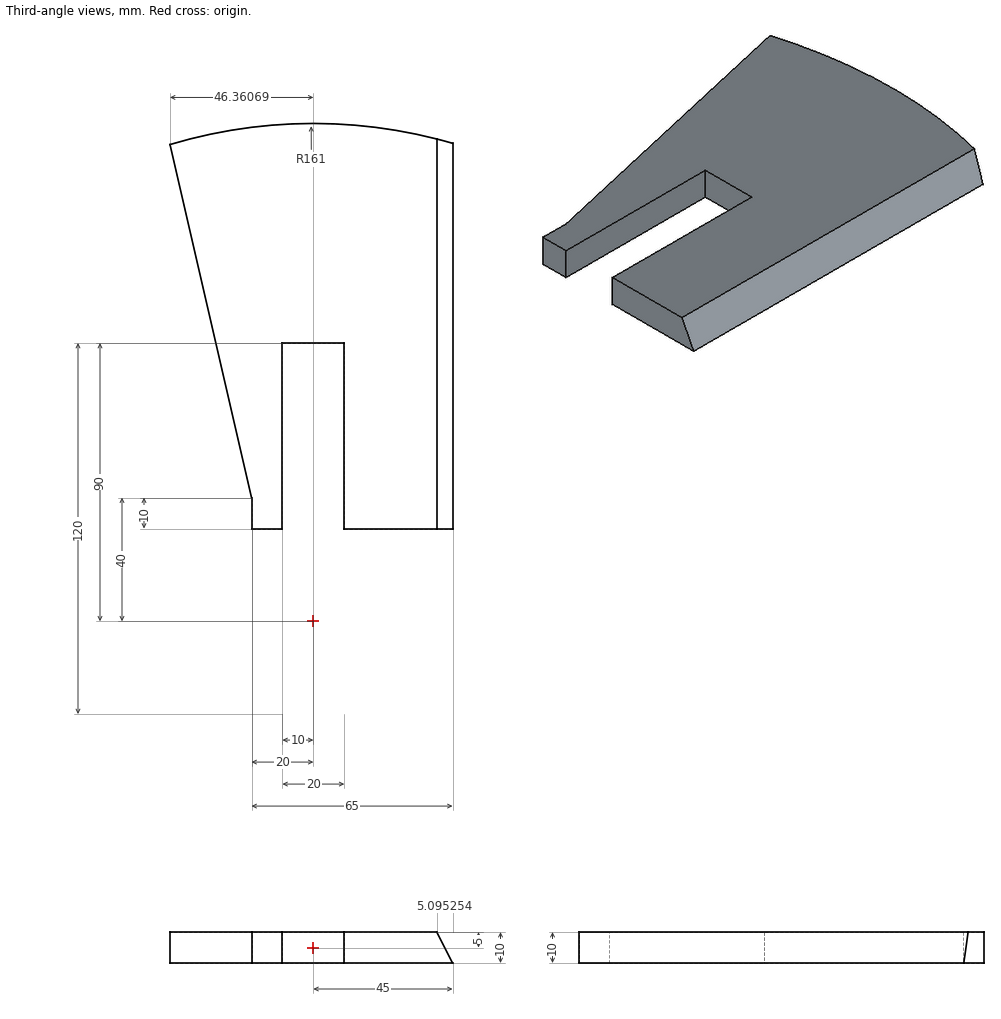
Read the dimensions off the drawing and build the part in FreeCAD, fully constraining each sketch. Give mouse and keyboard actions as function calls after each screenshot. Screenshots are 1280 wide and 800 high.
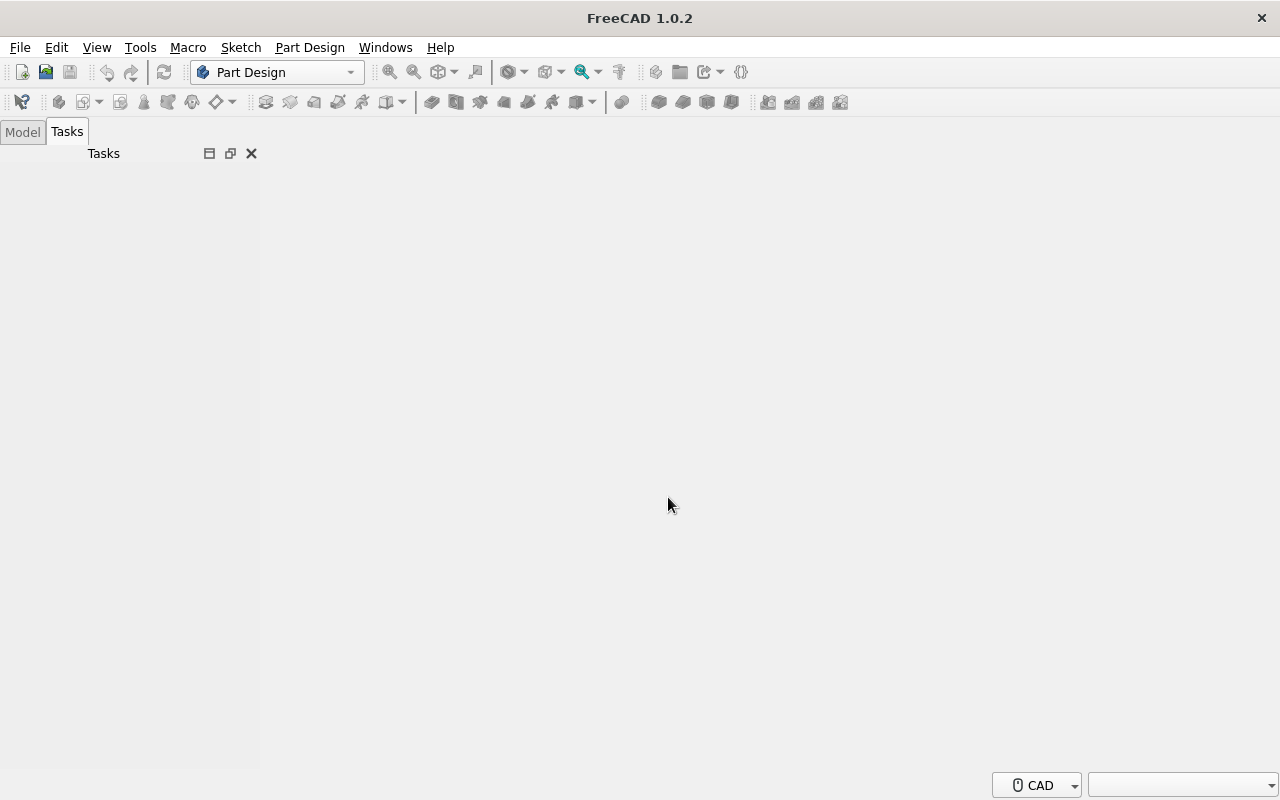
click(22, 72)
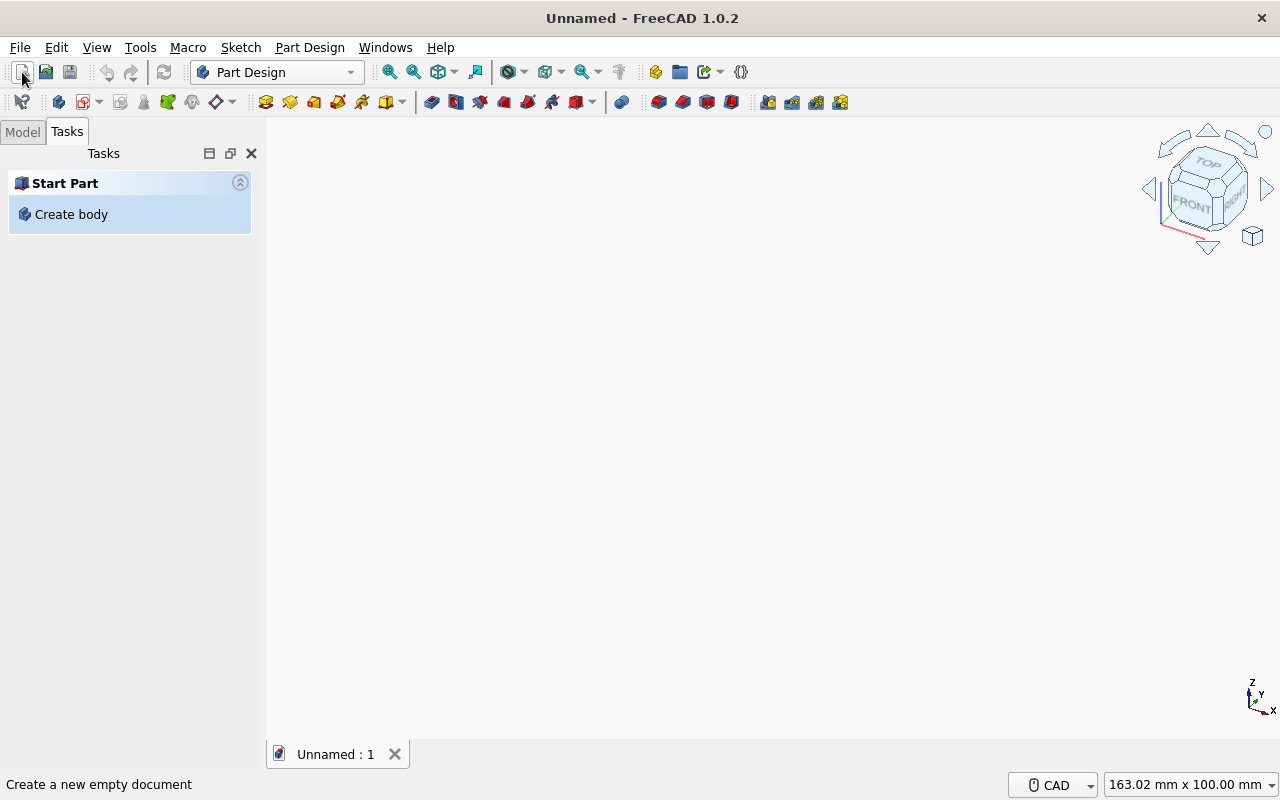
click(84, 102)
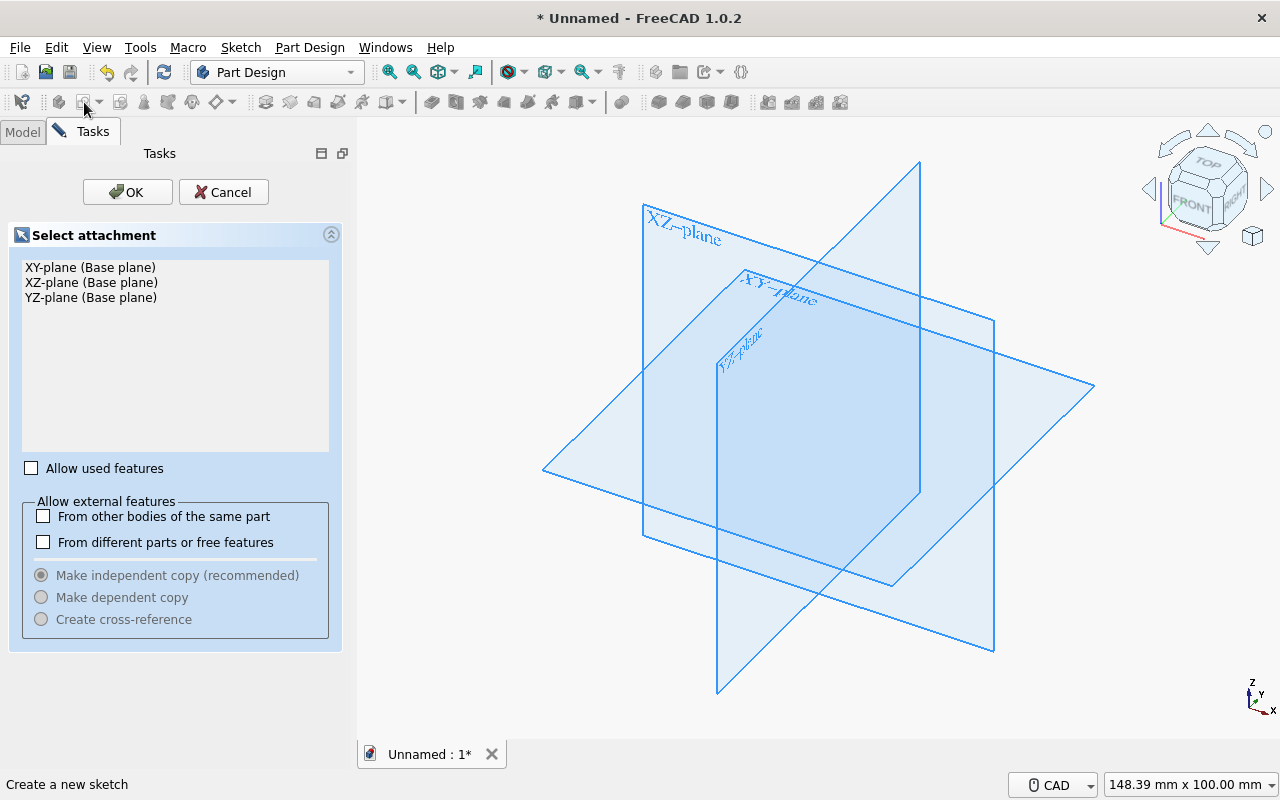
click(82, 268)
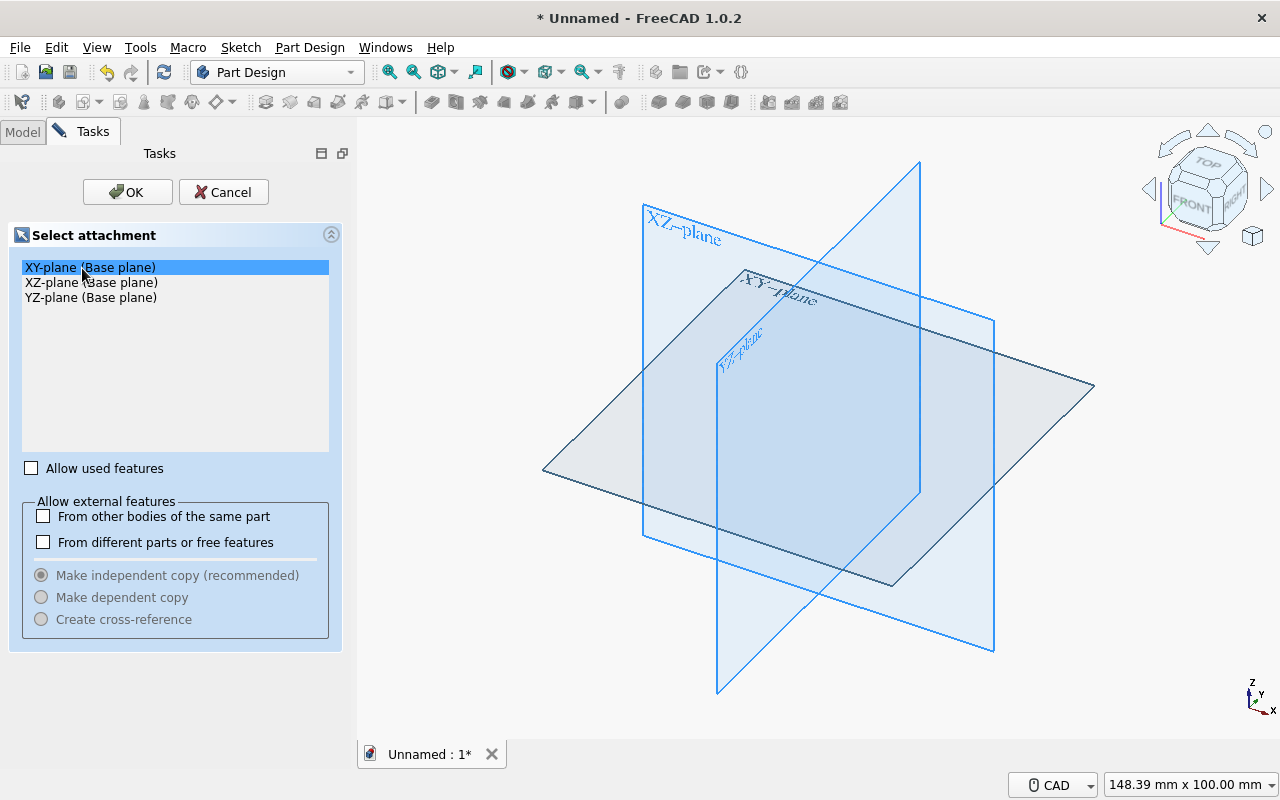
click(128, 192)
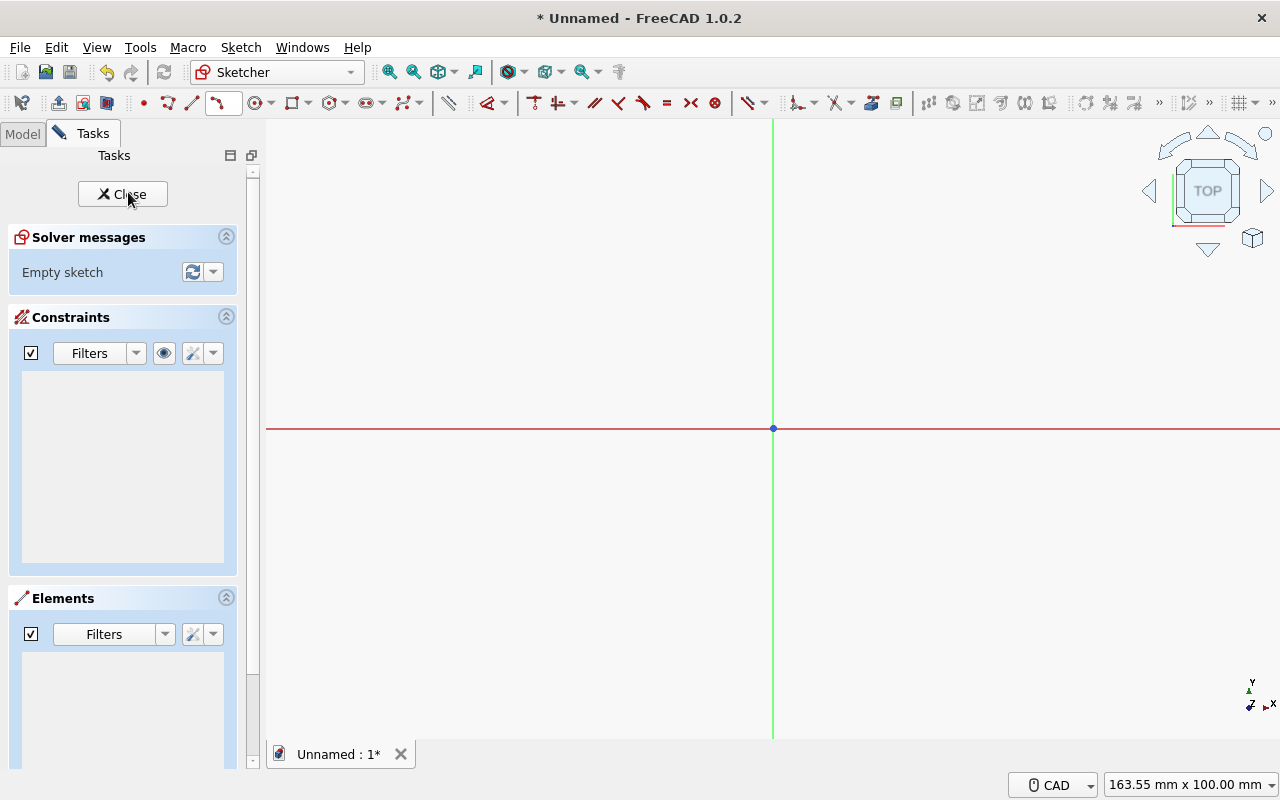
scroll(667, 711, down, 5)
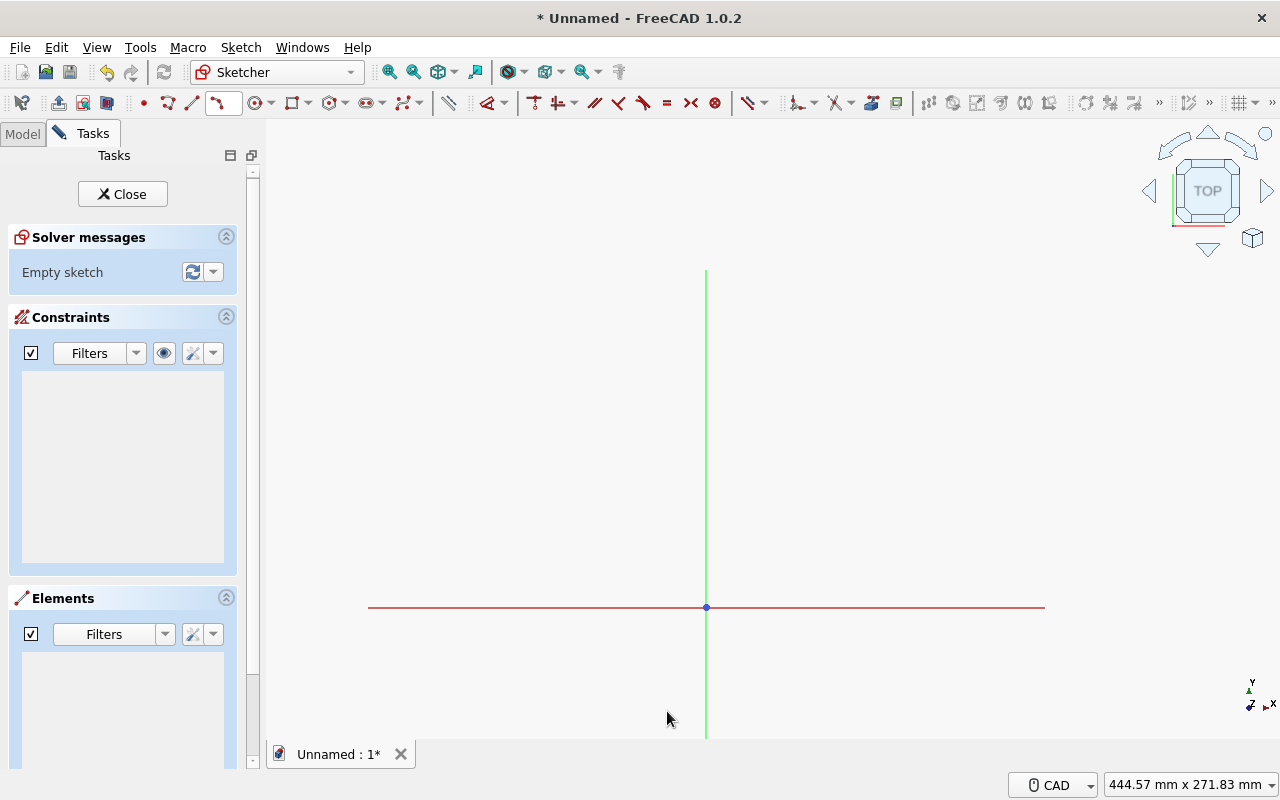
click(168, 104)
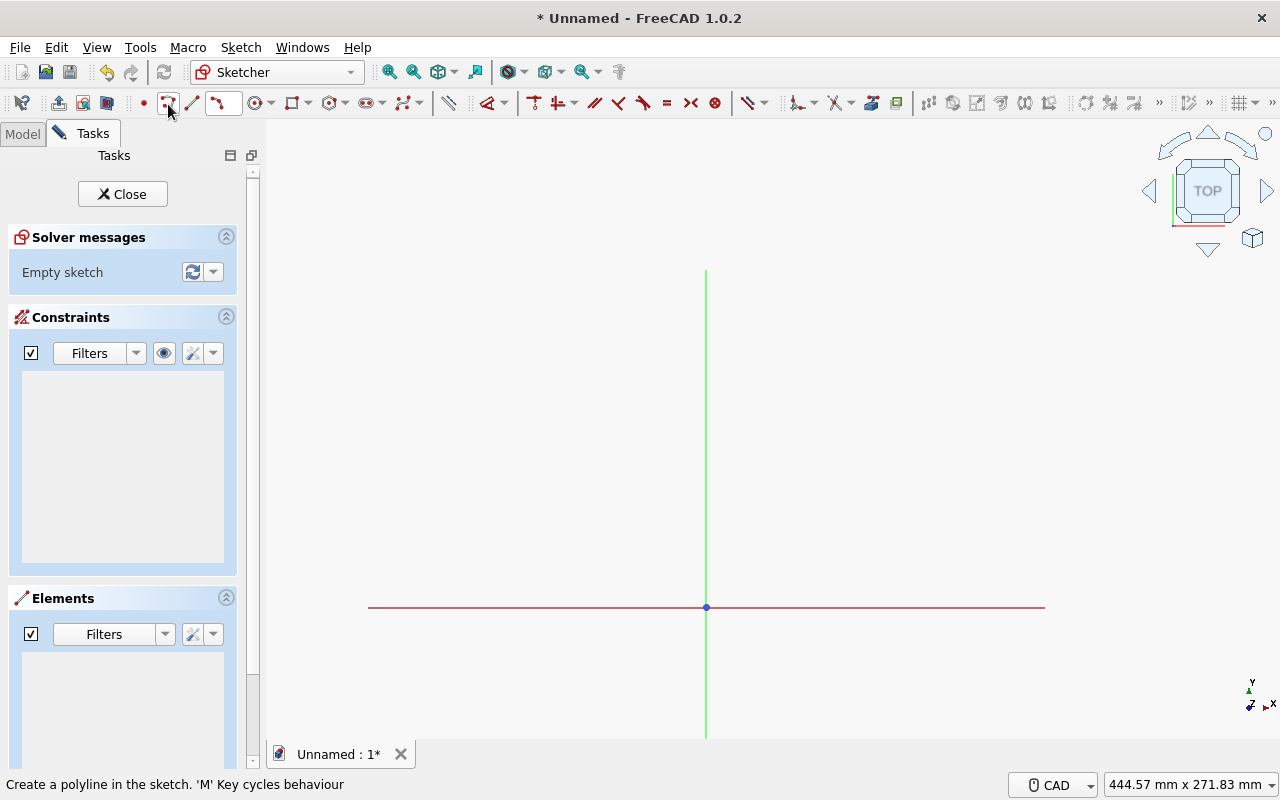
click(601, 256)
click(661, 517)
click(661, 539)
click(809, 539)
click(809, 255)
right_click(809, 255)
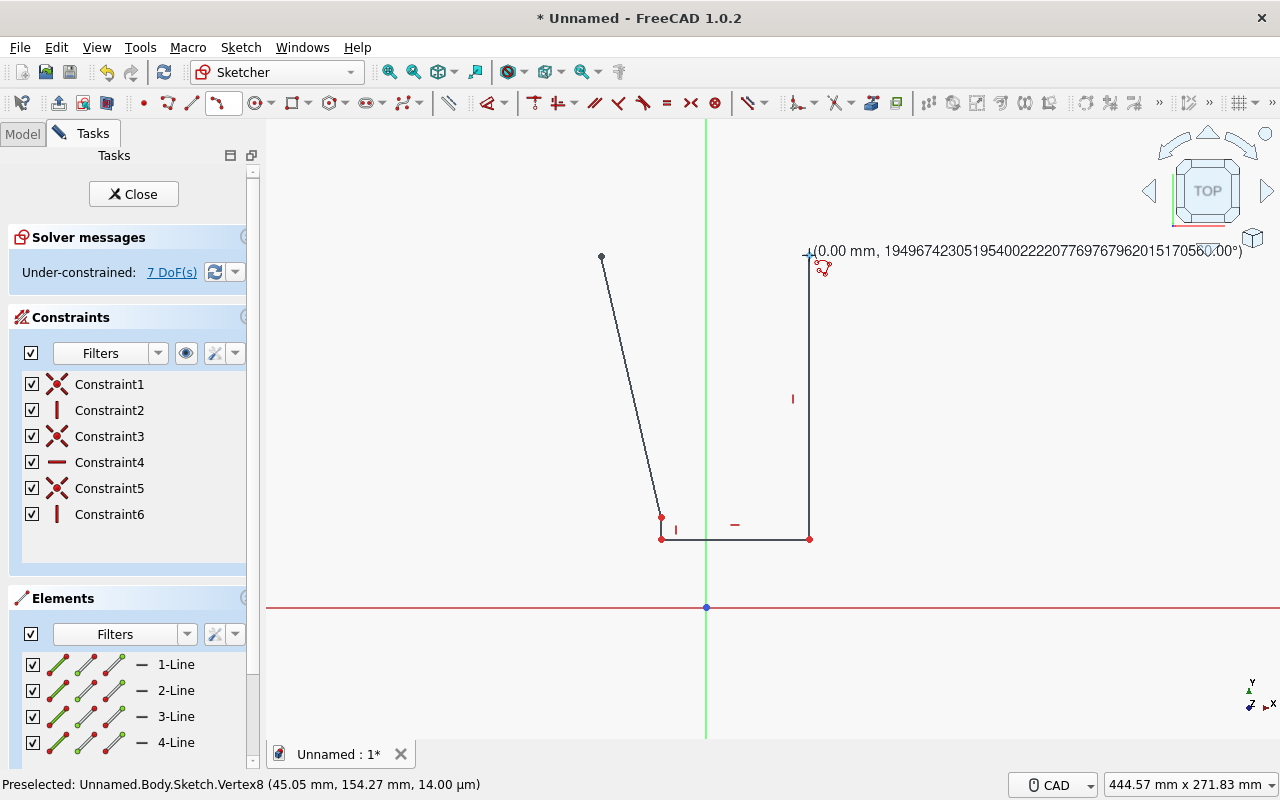
click(218, 104)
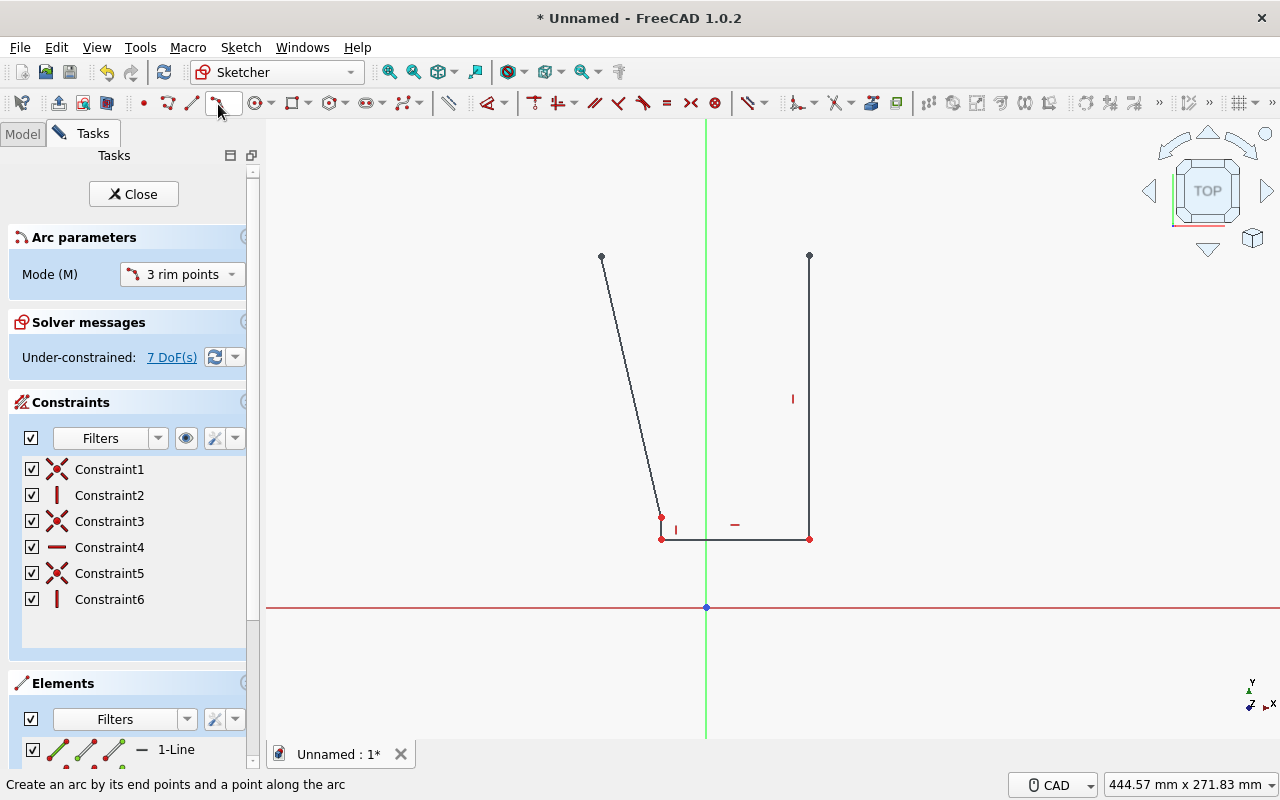
click(809, 256)
click(601, 257)
click(726, 241)
key(Escape)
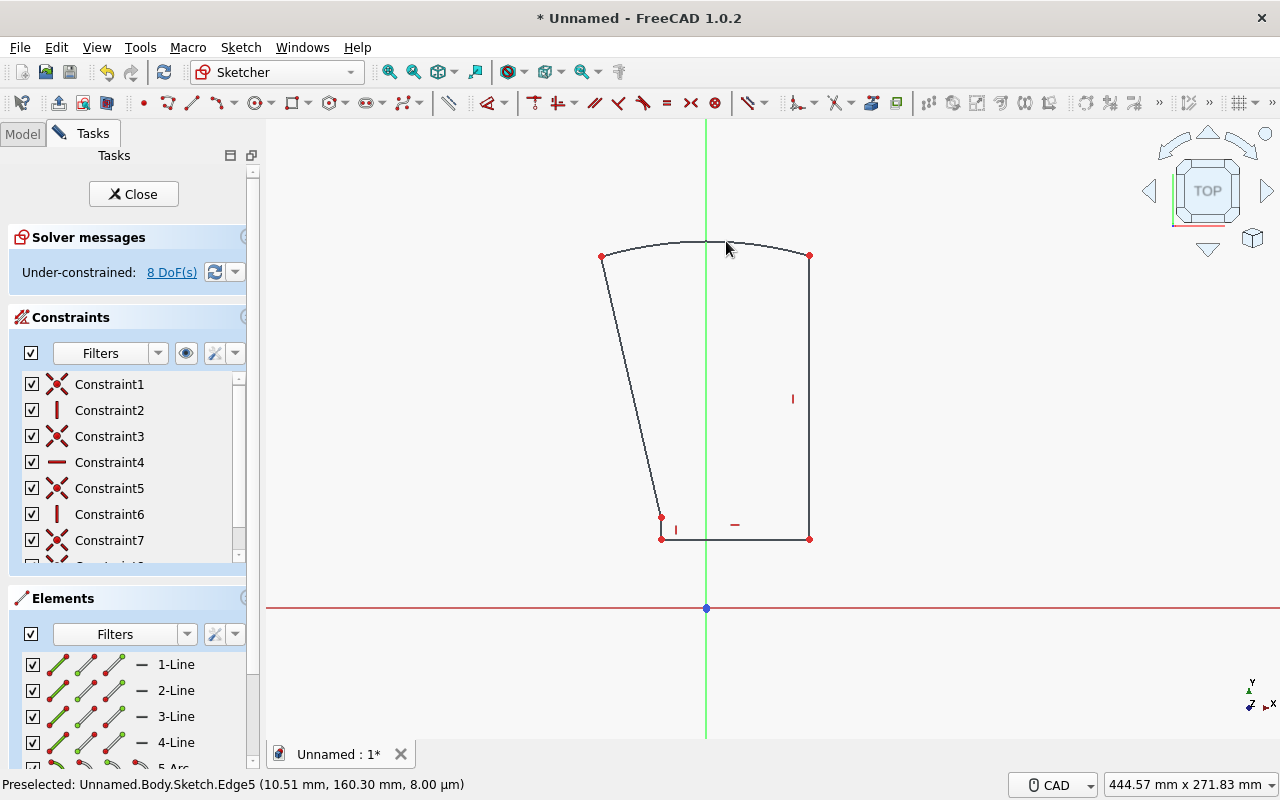
drag(696, 598, 717, 619)